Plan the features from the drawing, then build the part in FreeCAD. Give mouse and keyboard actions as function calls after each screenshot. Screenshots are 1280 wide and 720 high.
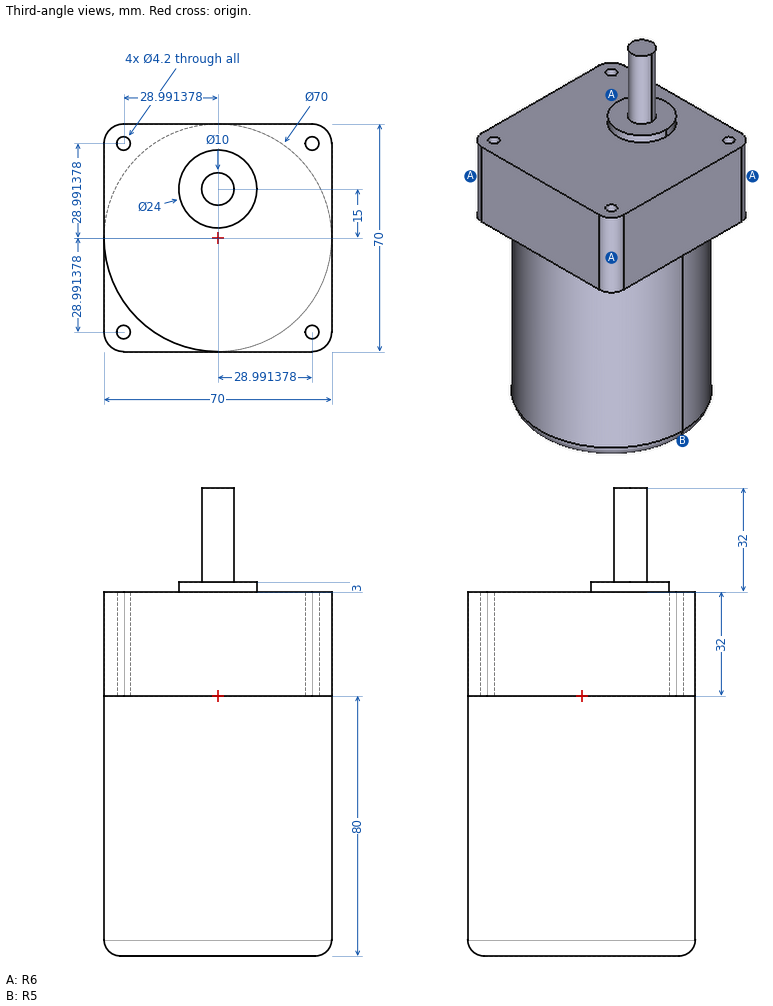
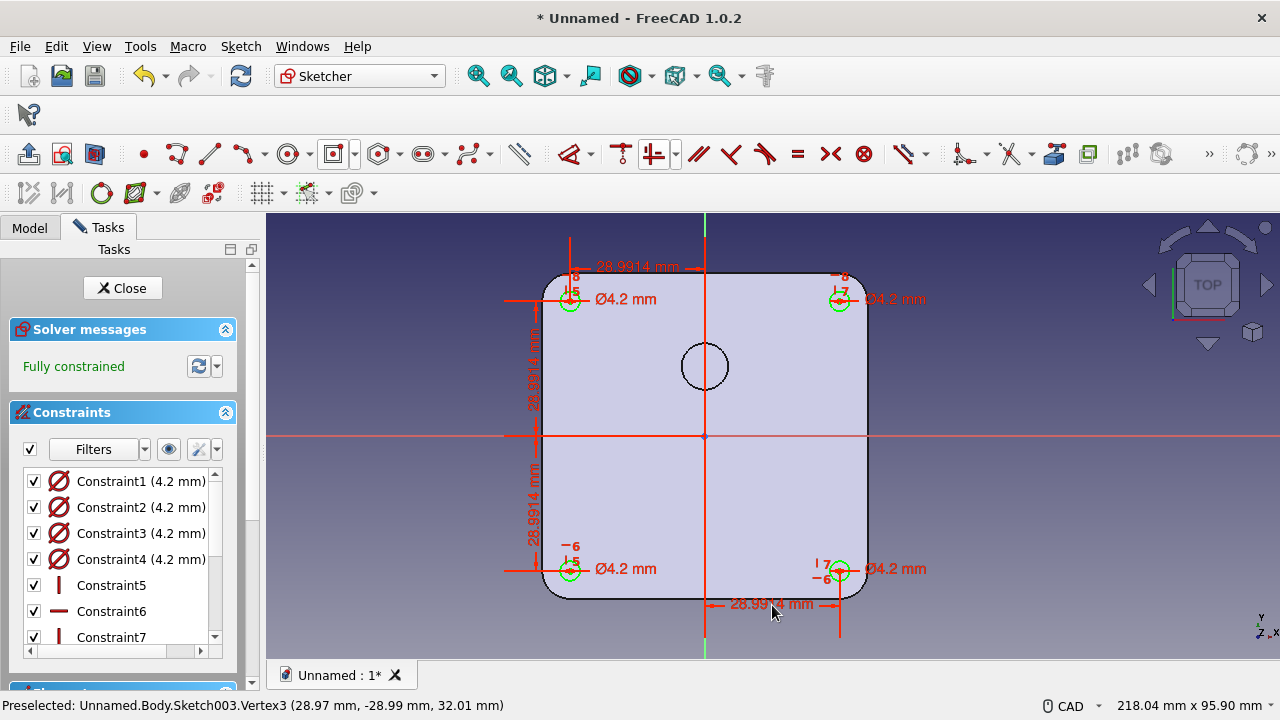
click(123, 288)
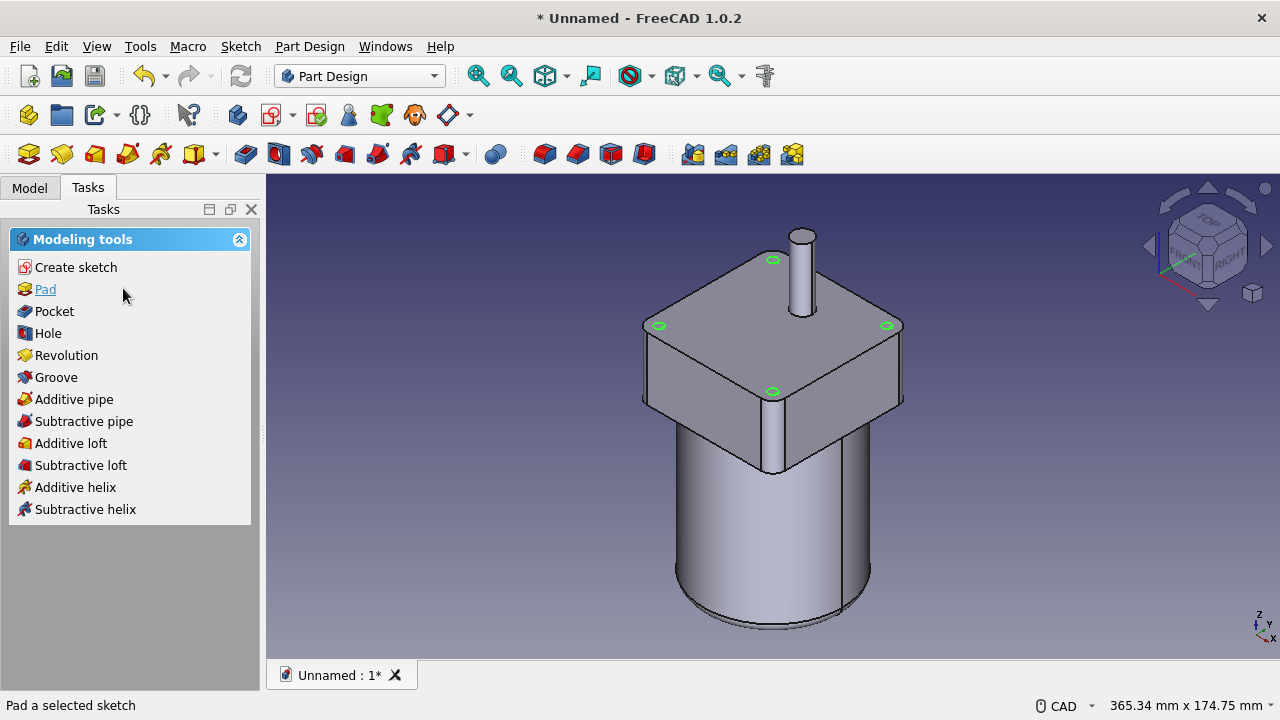
click(279, 154)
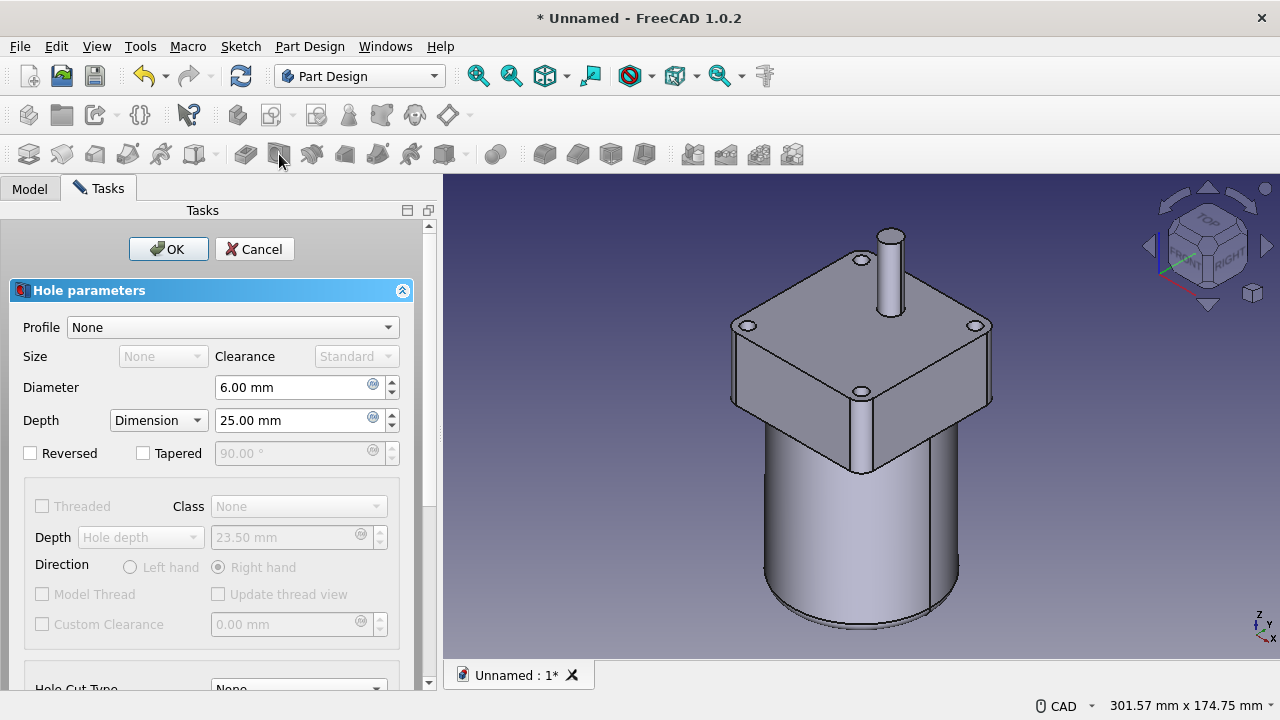
triple_click(300, 388)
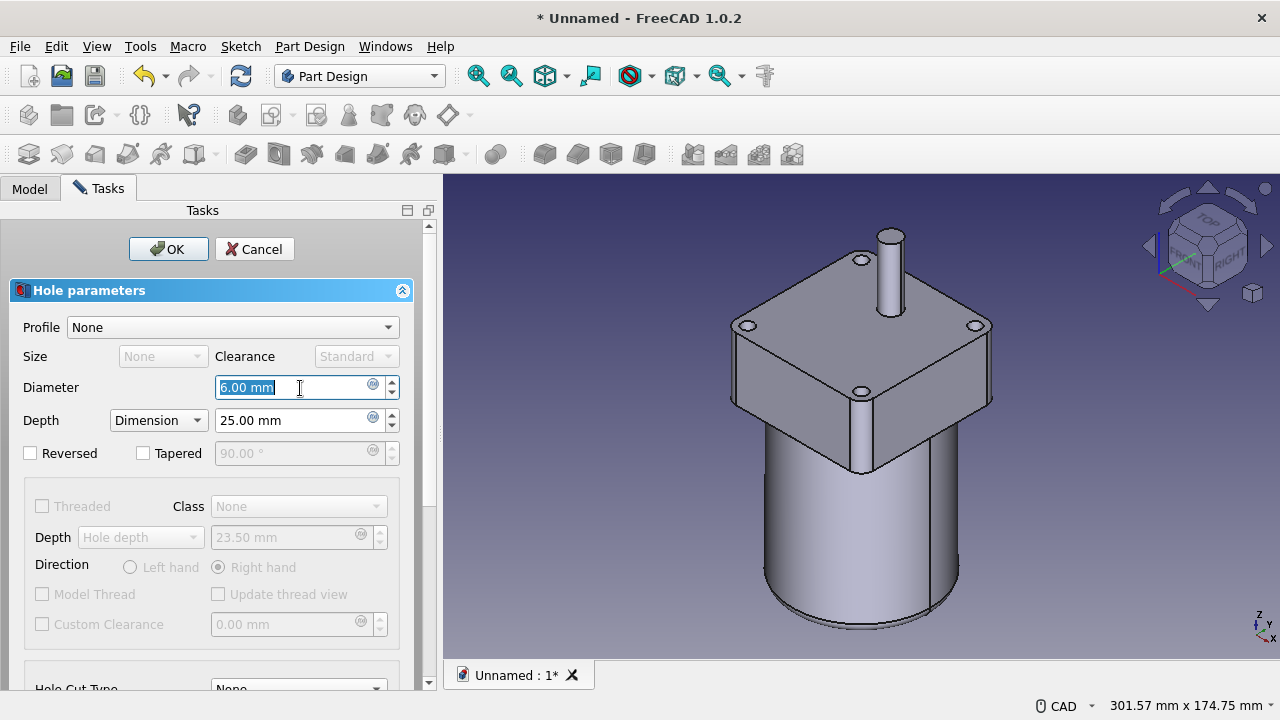
text(4.2)
key(Tab)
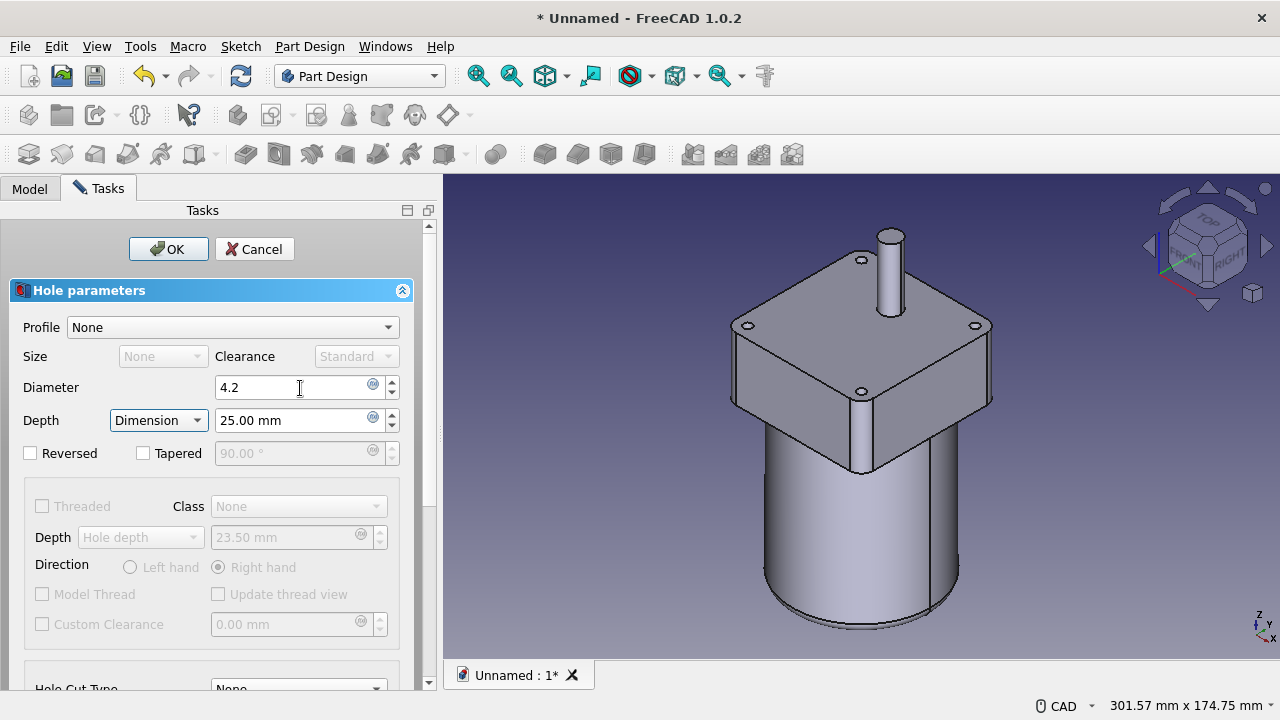
click(160, 420)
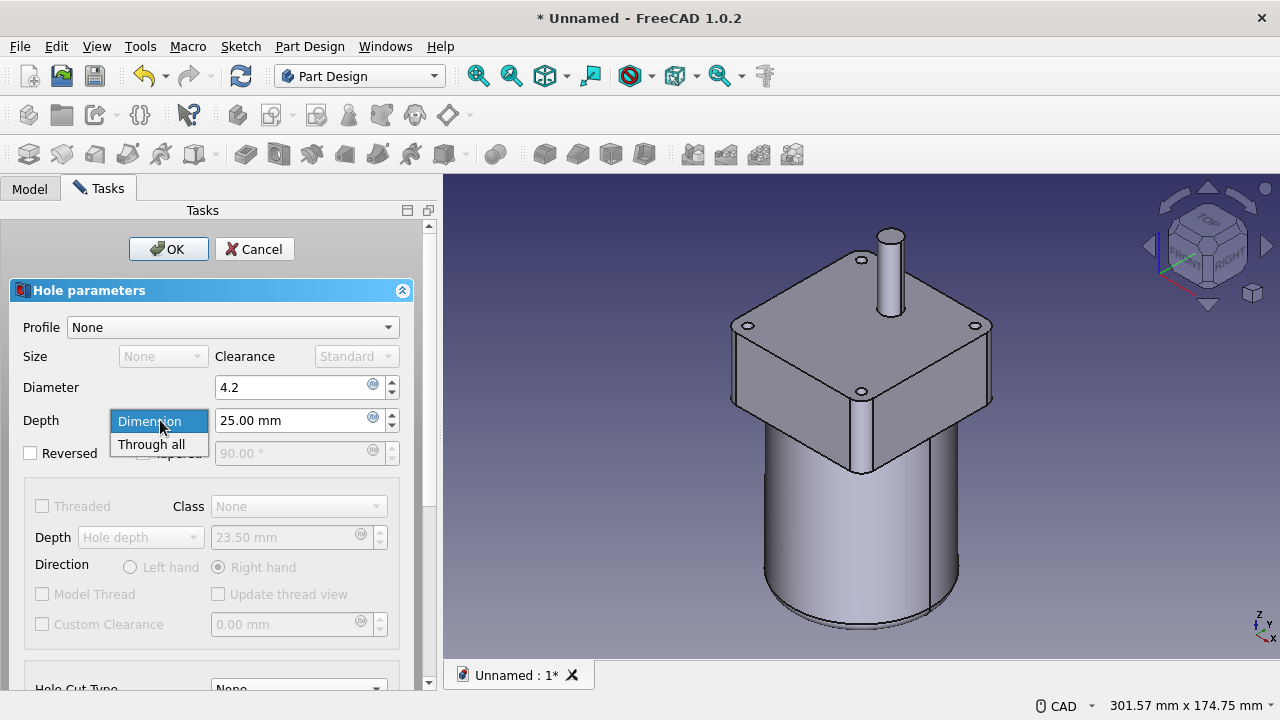
click(158, 444)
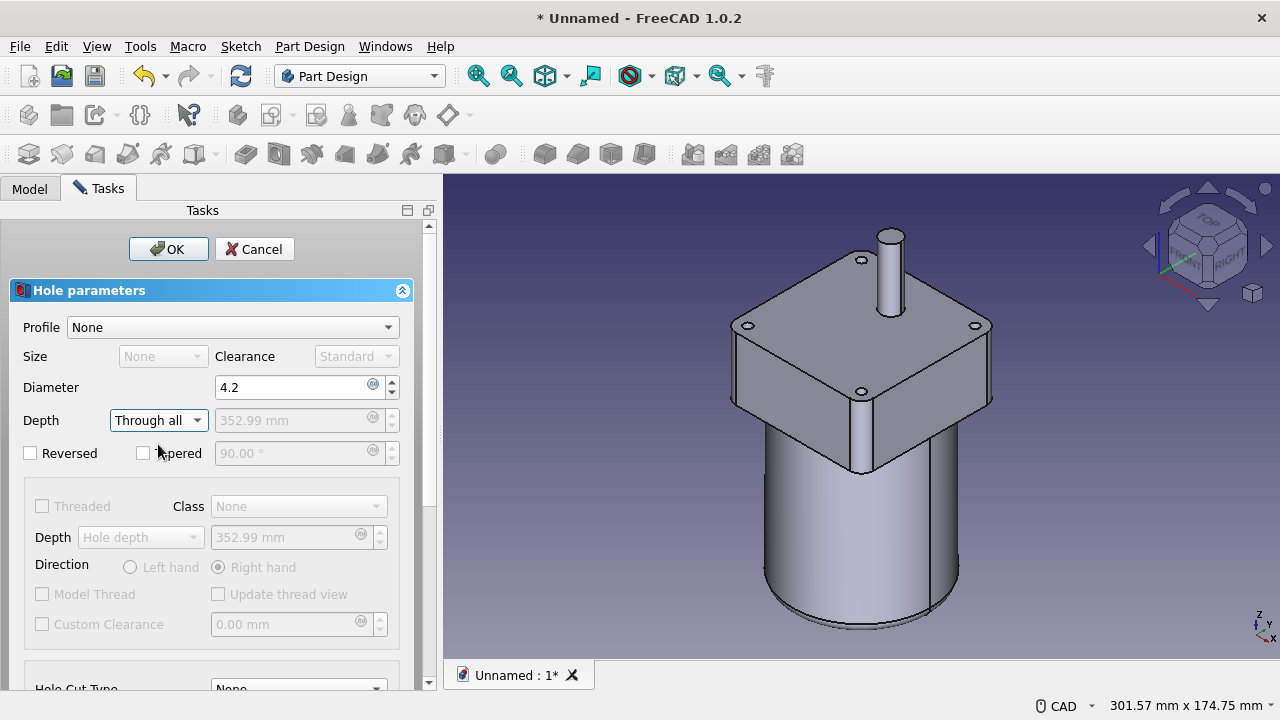
click(169, 249)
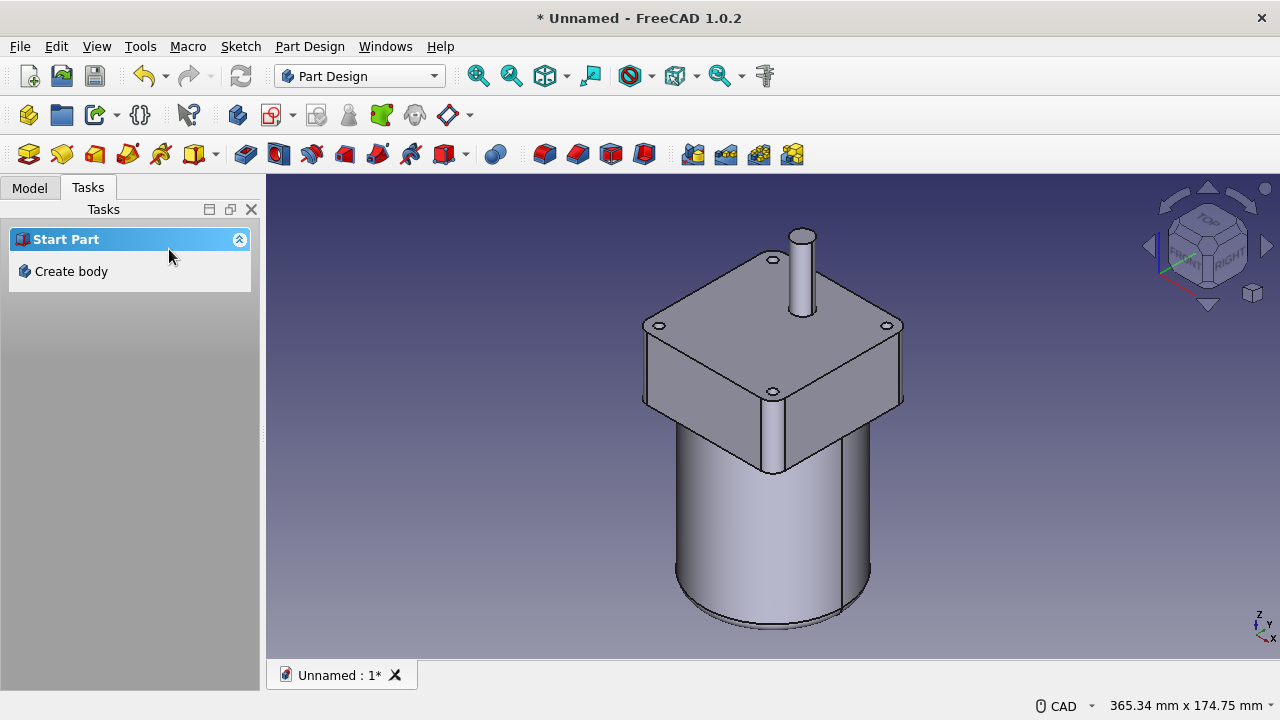
key(v)
key(f)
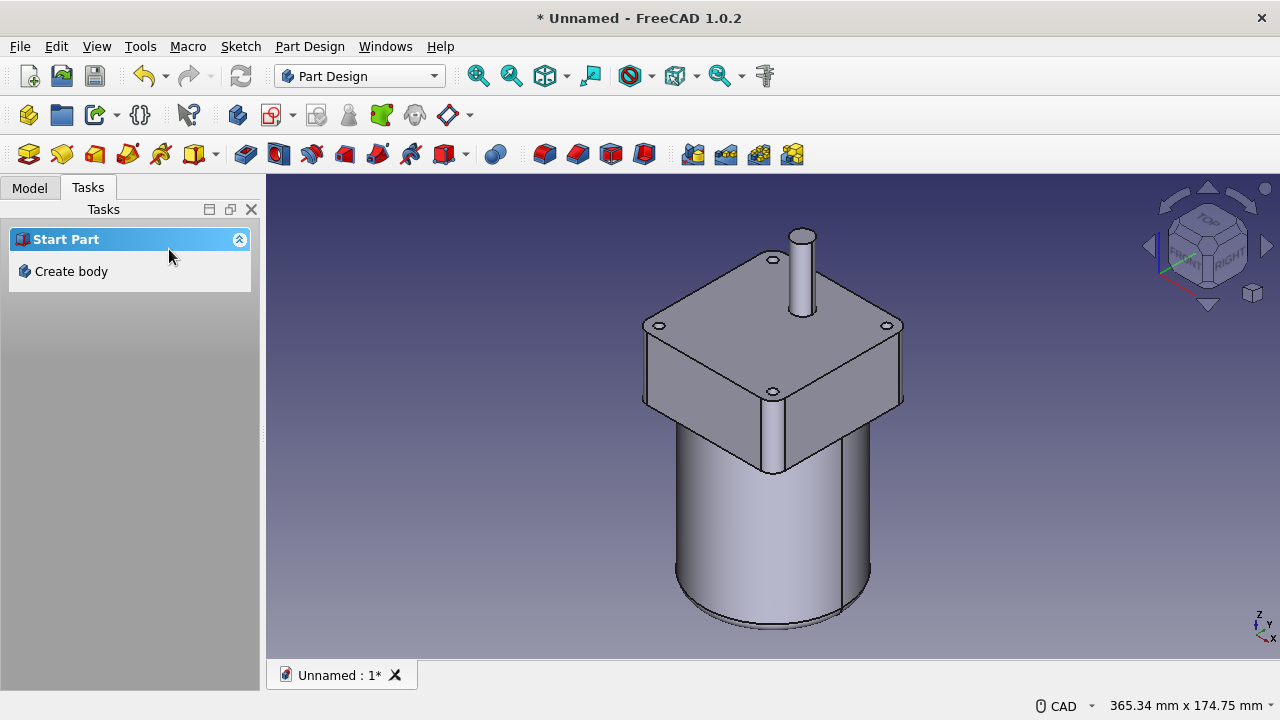
click(773, 348)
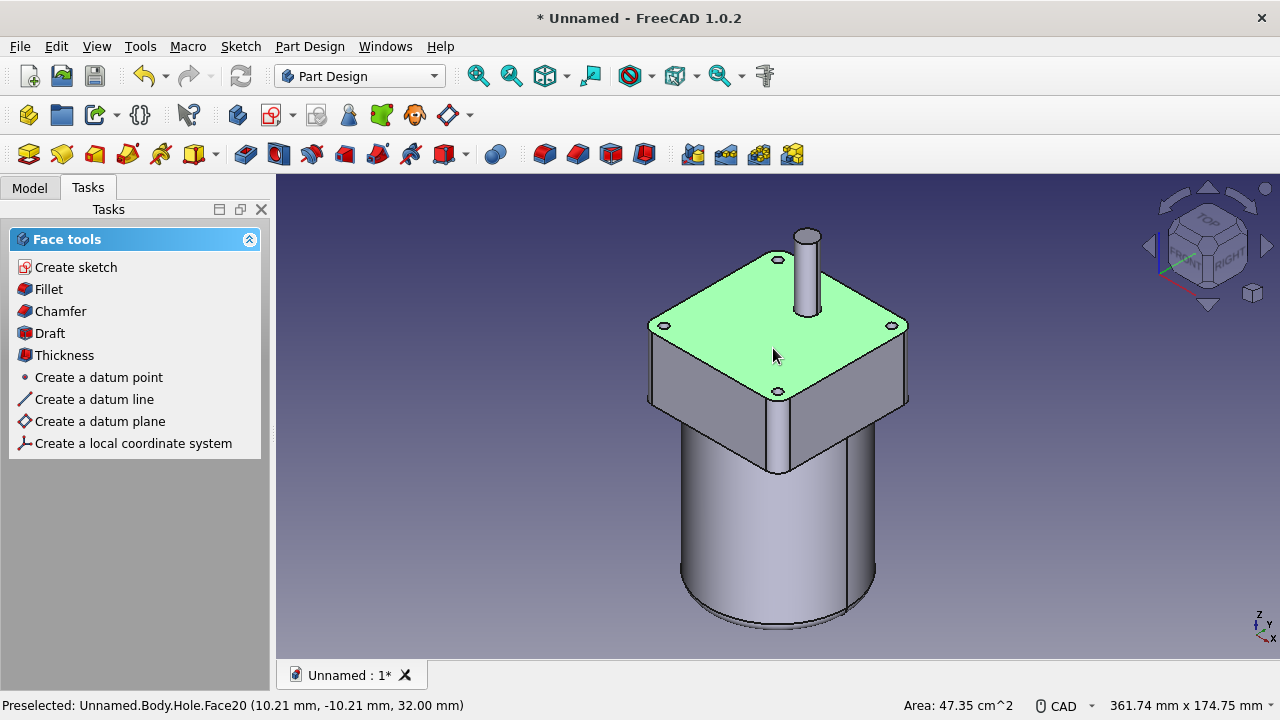
click(270, 116)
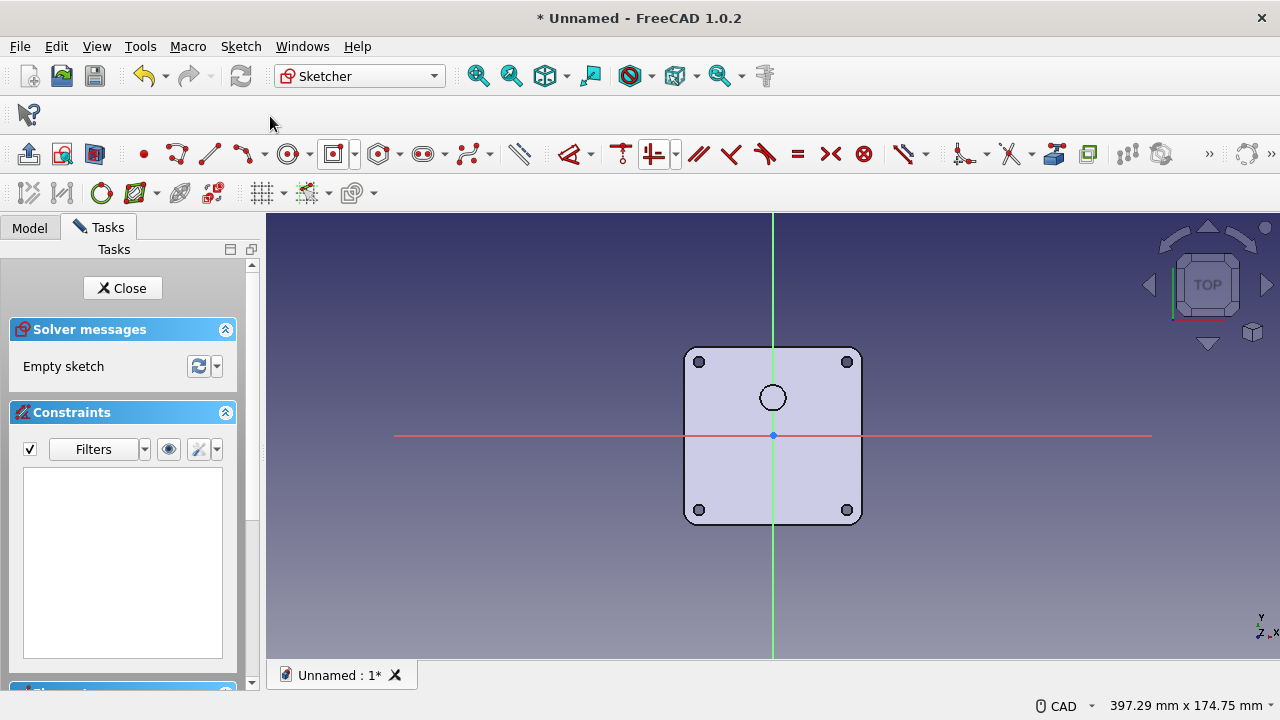
click(95, 154)